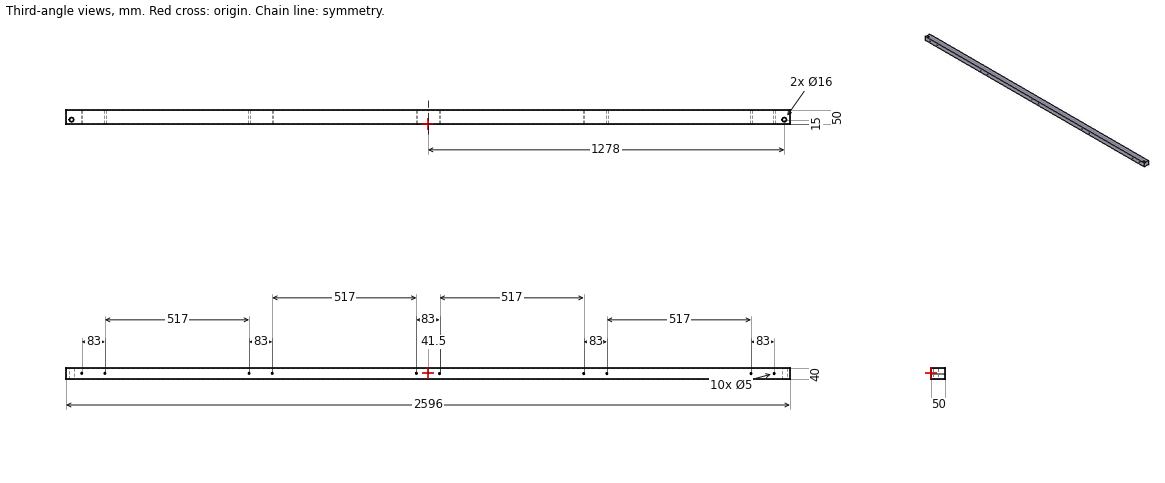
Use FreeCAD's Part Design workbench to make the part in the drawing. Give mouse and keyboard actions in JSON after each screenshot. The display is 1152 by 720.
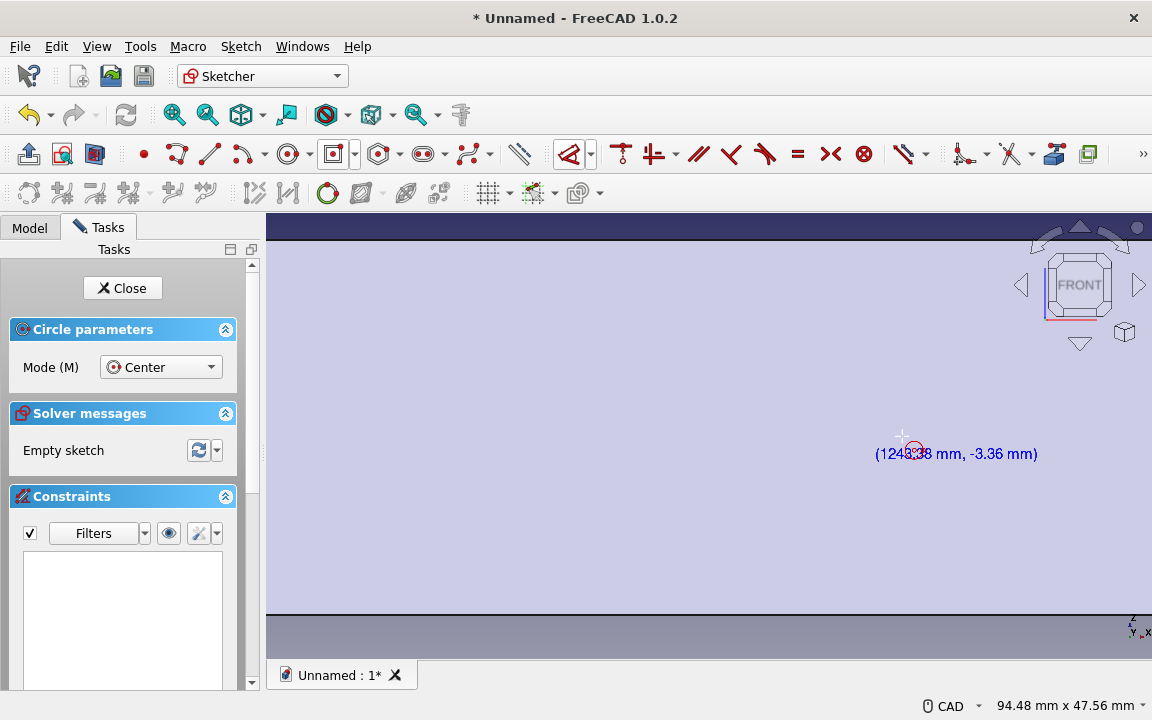
{"action": "scroll", "coordinate": [962, 436], "scroll_direction": "down", "scroll_amount": 18}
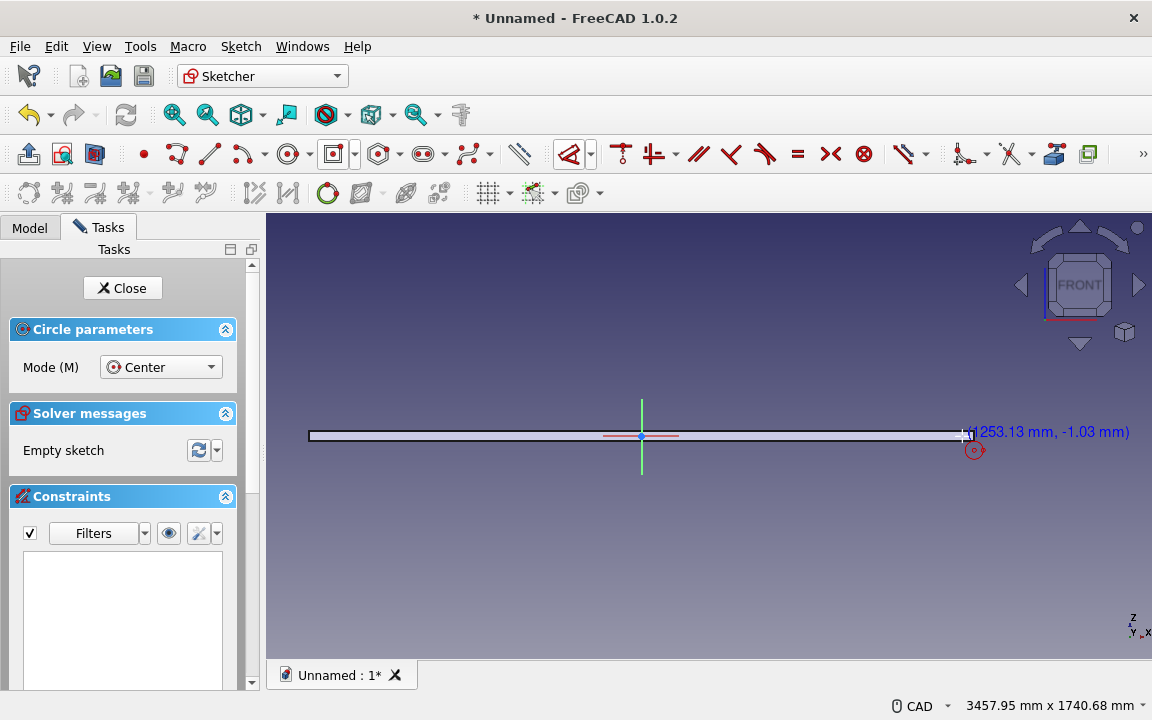
{"action": "left_click", "coordinate": [960, 436]}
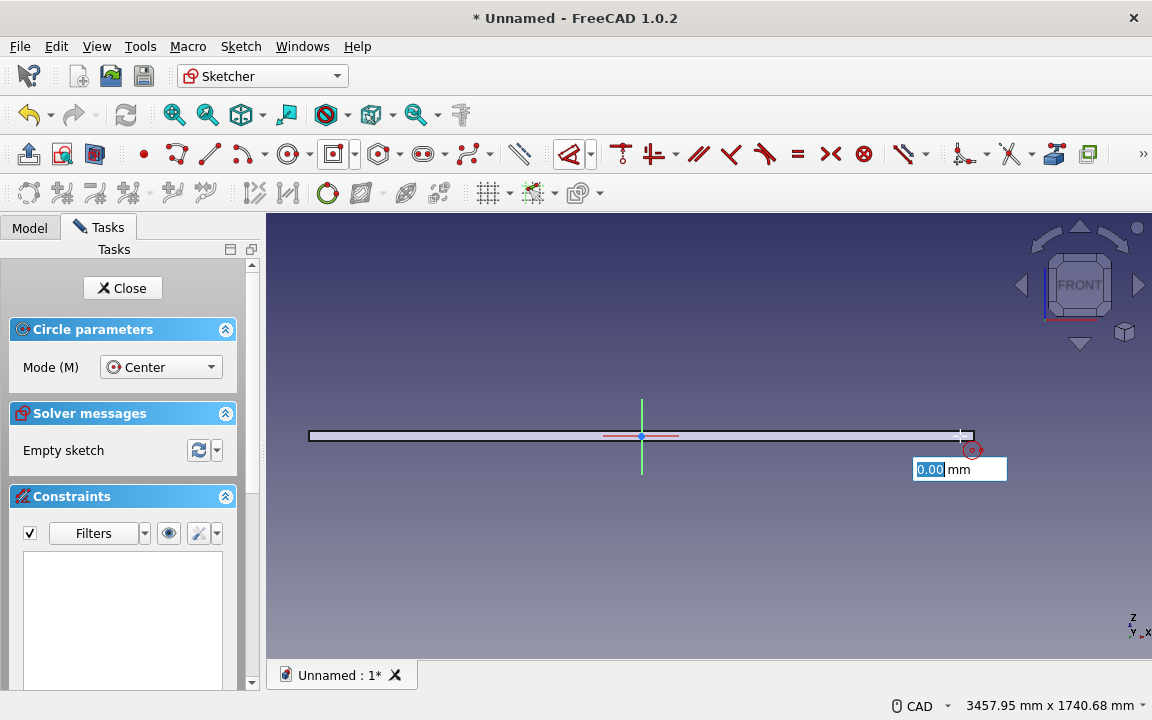
{"action": "scroll", "coordinate": [960, 437], "scroll_direction": "up", "scroll_amount": 17}
{"action": "mouse_move", "coordinate": [924, 418]}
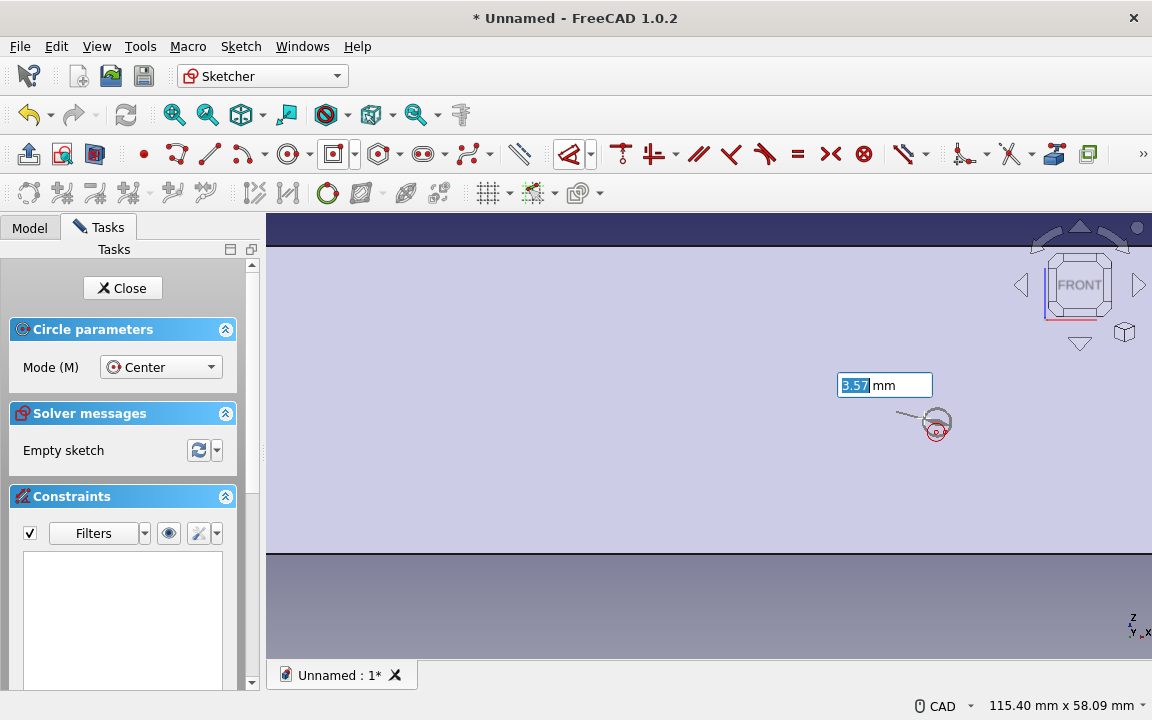
{"action": "type", "text": "5"}
{"action": "key", "text": "Return"}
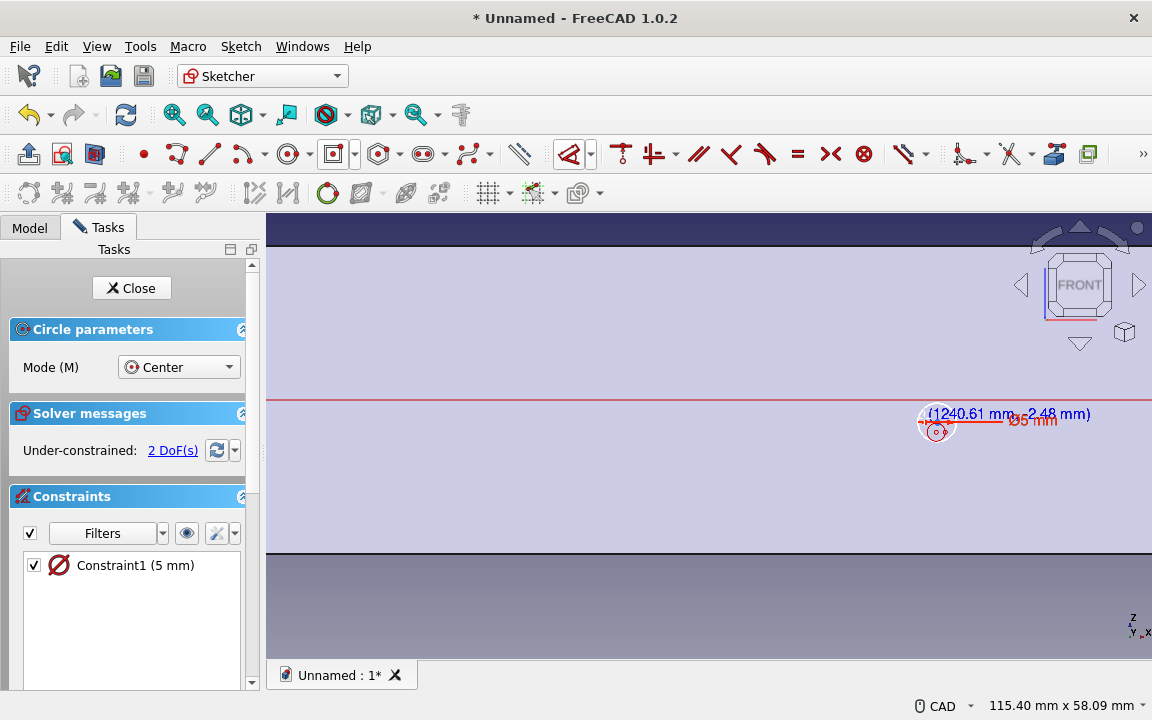
{"action": "scroll", "coordinate": [960, 437], "scroll_direction": "down", "scroll_amount": 17}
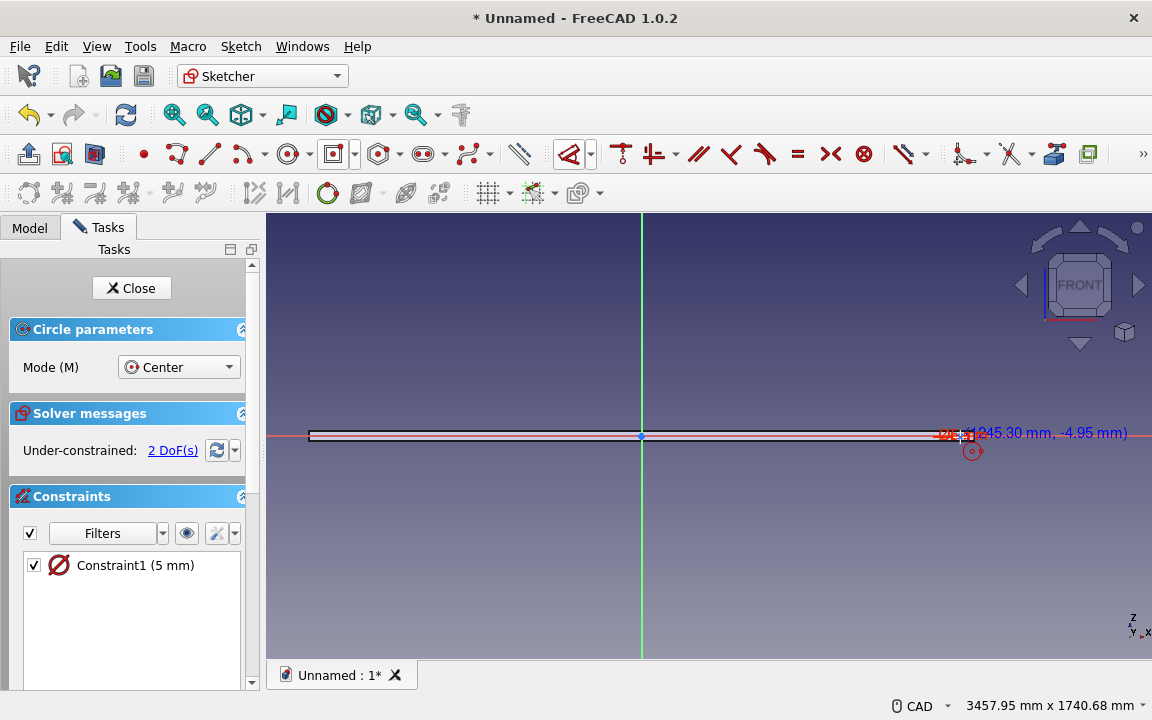
{"action": "scroll", "coordinate": [939, 436], "scroll_direction": "up", "scroll_amount": 18}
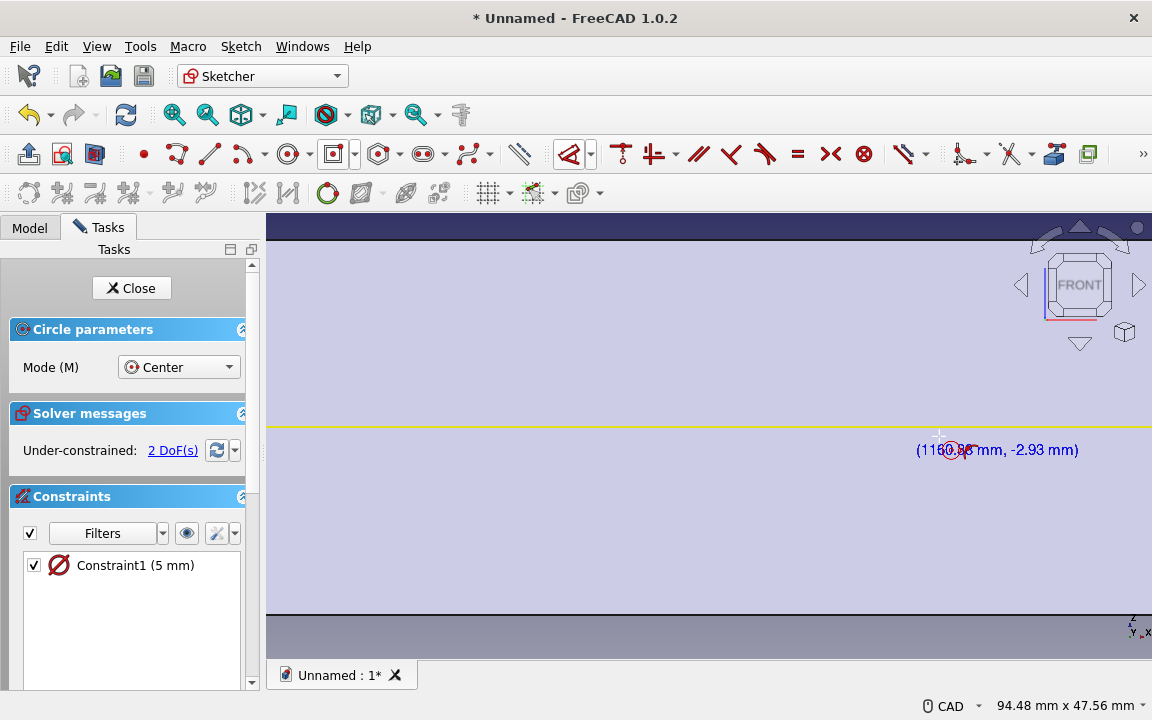
{"action": "scroll", "coordinate": [939, 436], "scroll_direction": "down", "scroll_amount": 18}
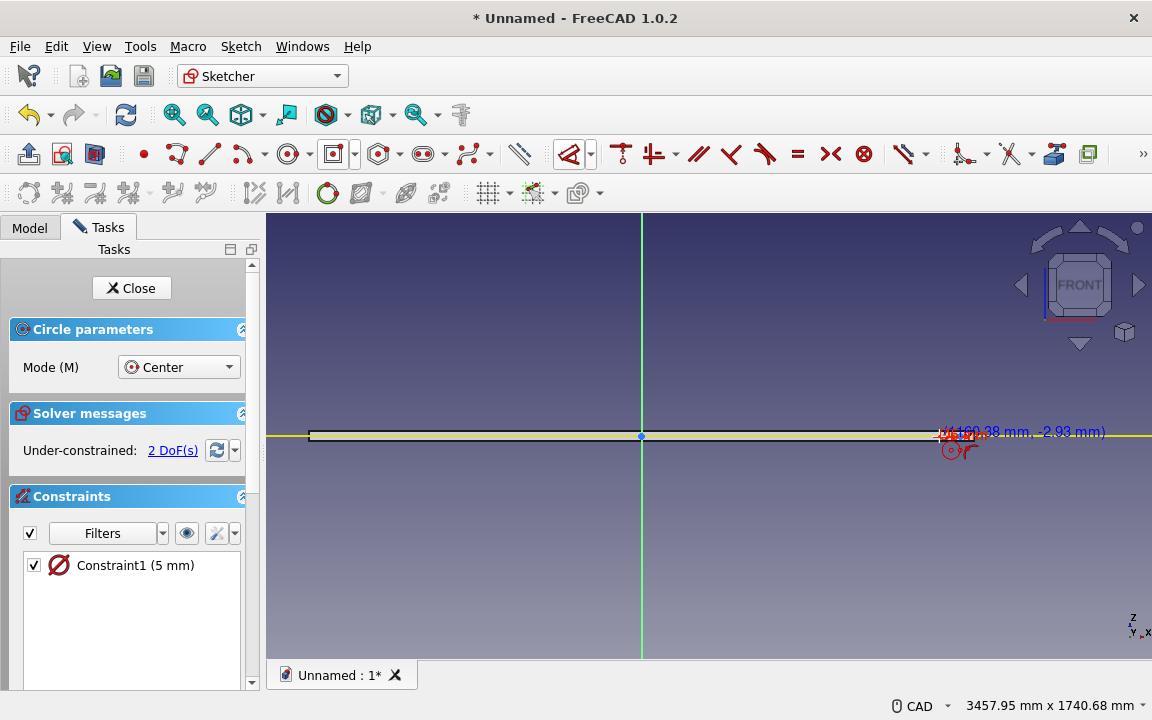
{"action": "left_click", "coordinate": [939, 436]}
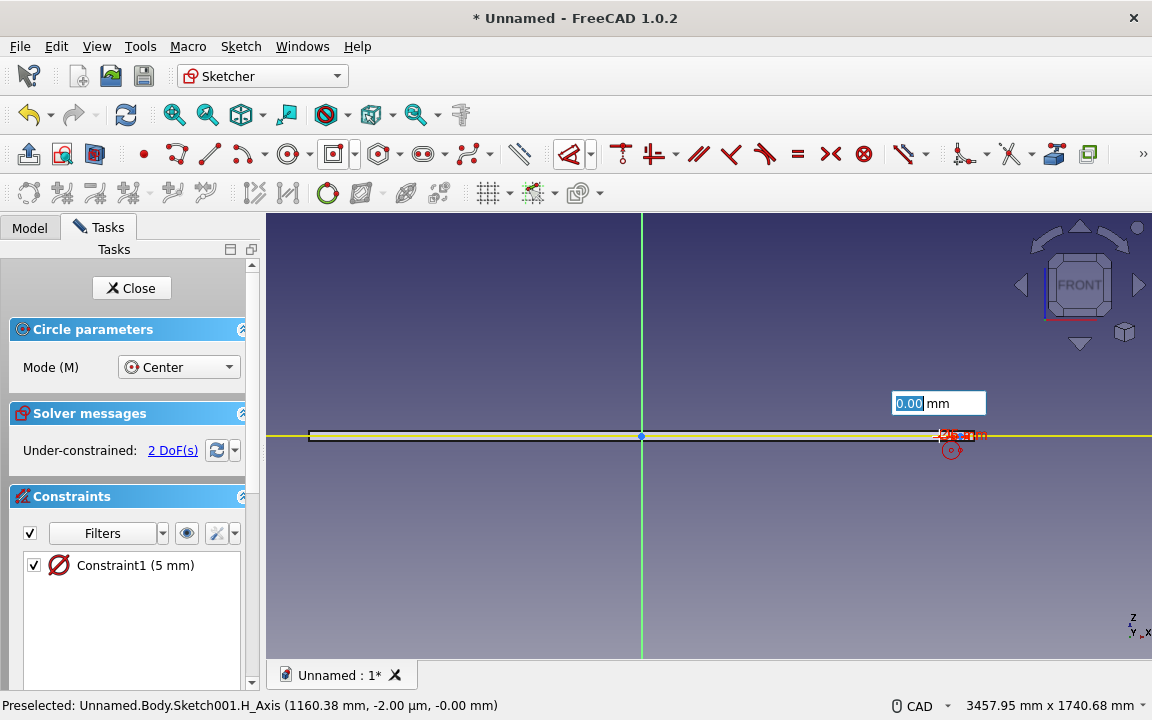
{"action": "scroll", "coordinate": [938, 437], "scroll_direction": "up", "scroll_amount": 17}
{"action": "mouse_move", "coordinate": [925, 418]}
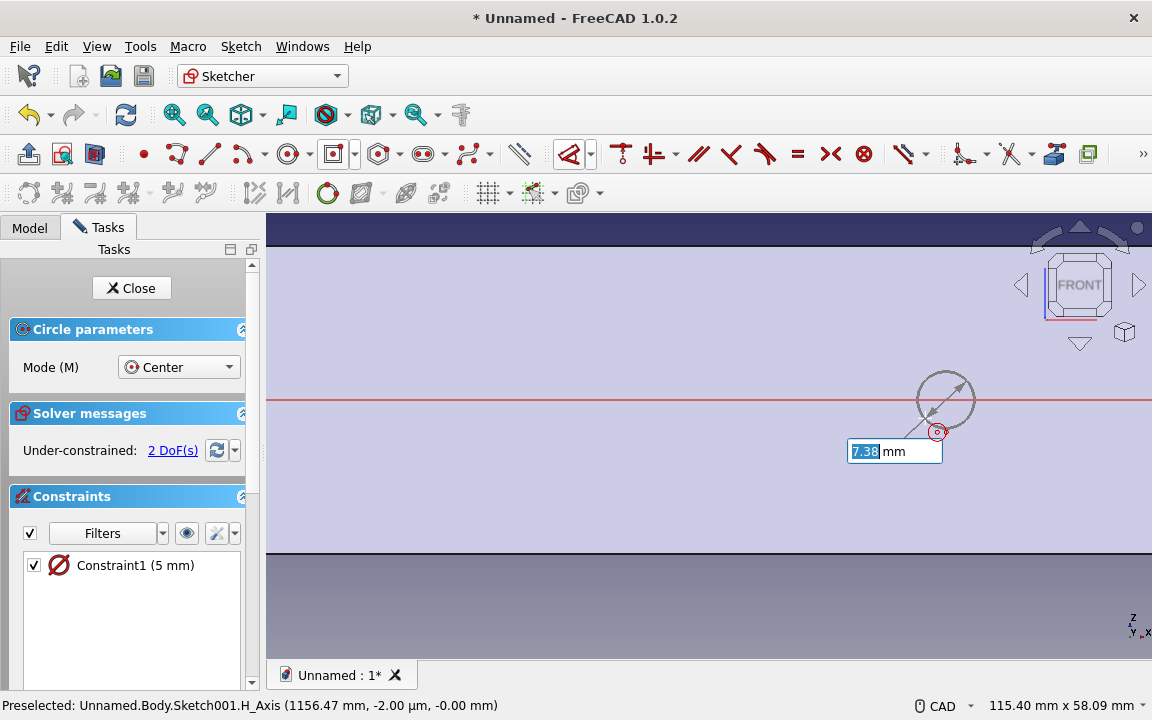
{"action": "type", "text": "5"}
{"action": "key", "text": "Return"}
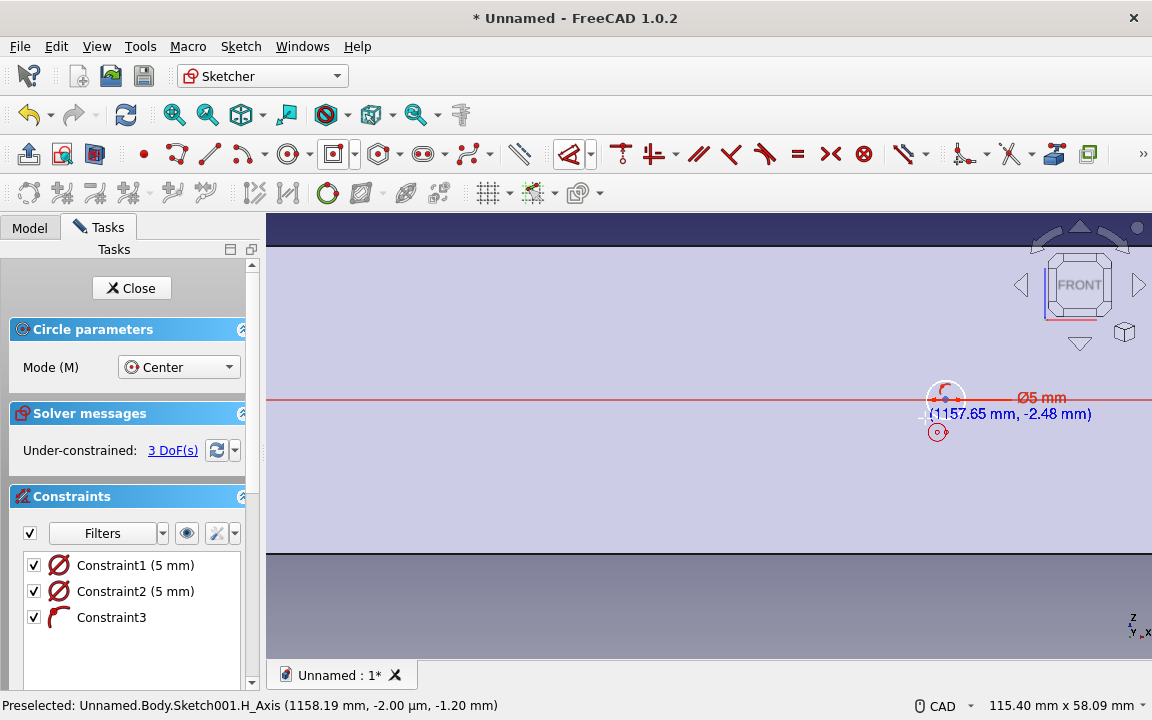
{"action": "scroll", "coordinate": [938, 437], "scroll_direction": "down", "scroll_amount": 17}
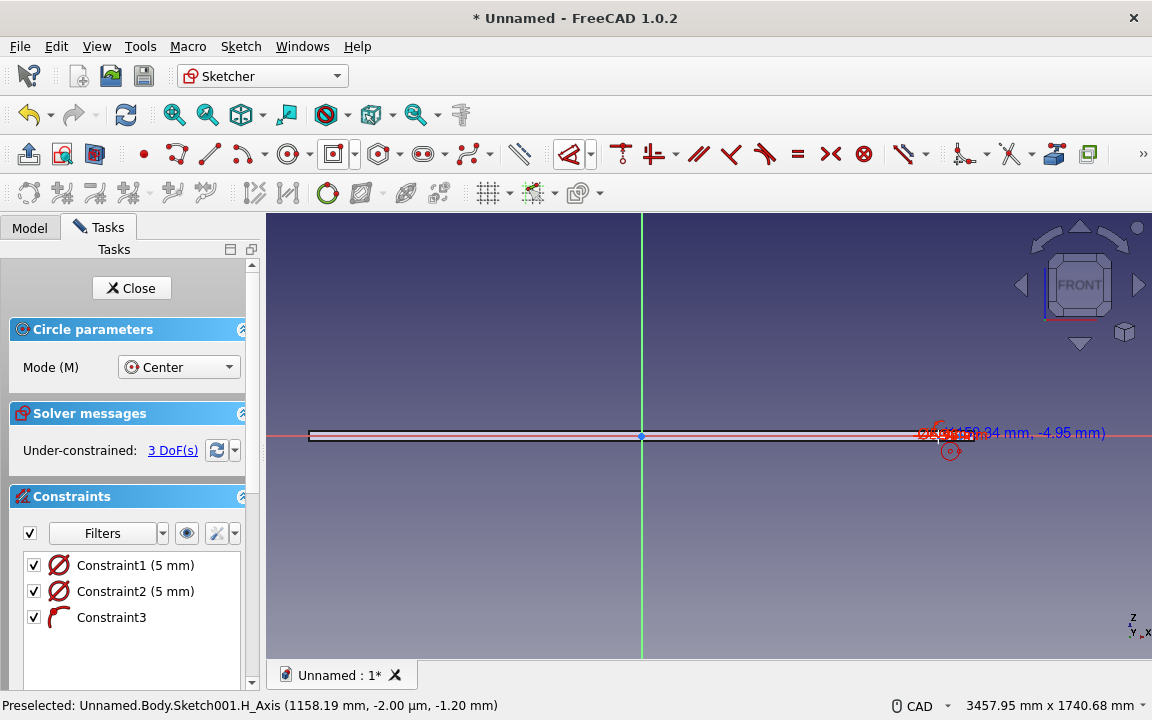
{"action": "scroll", "coordinate": [806, 436], "scroll_direction": "up", "scroll_amount": 18}